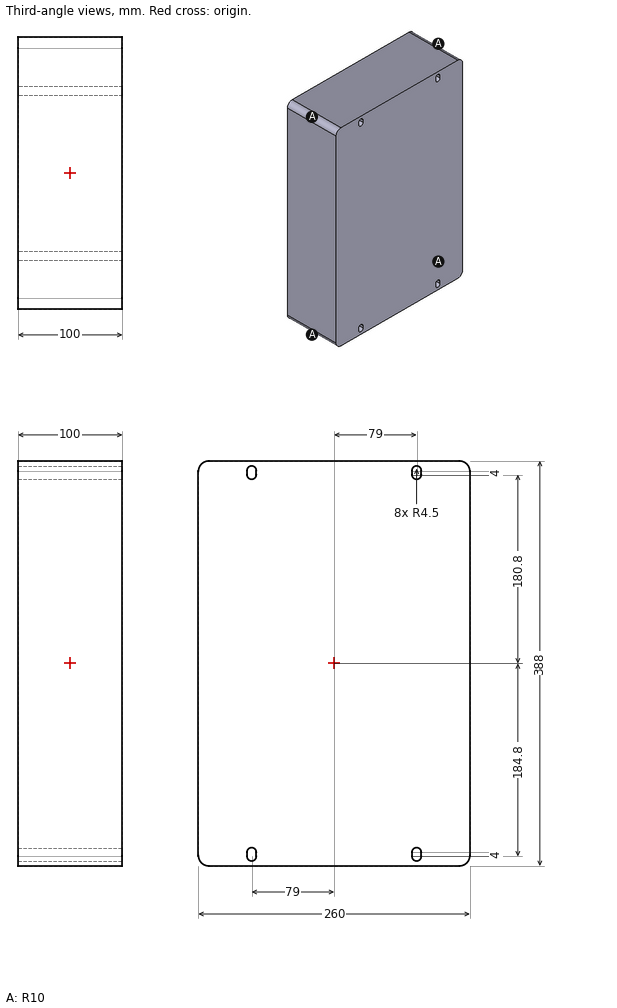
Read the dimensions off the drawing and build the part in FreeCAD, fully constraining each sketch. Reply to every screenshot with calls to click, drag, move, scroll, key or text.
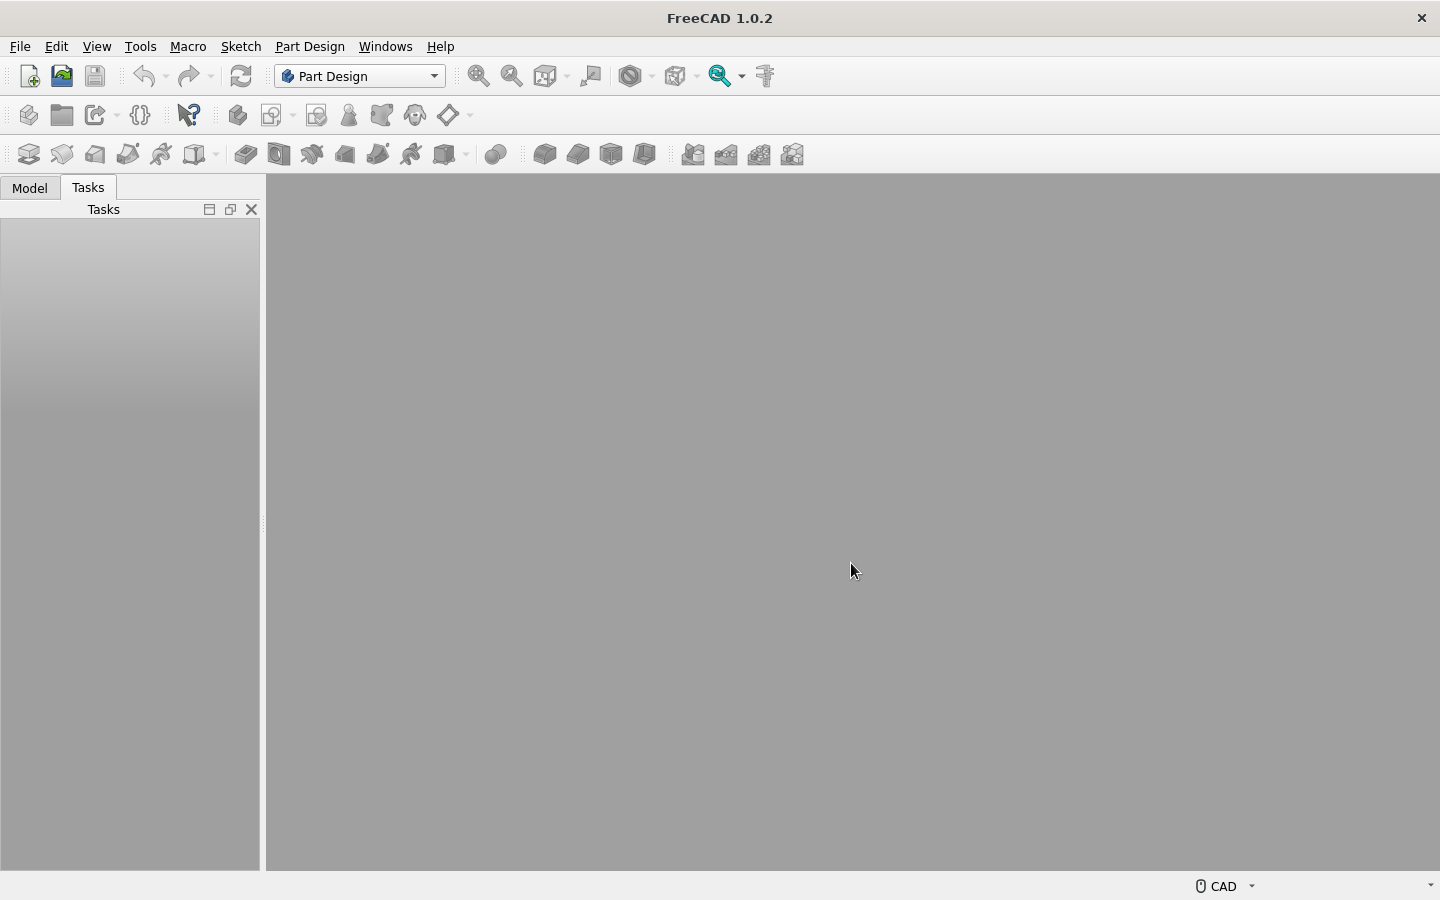
click(29, 76)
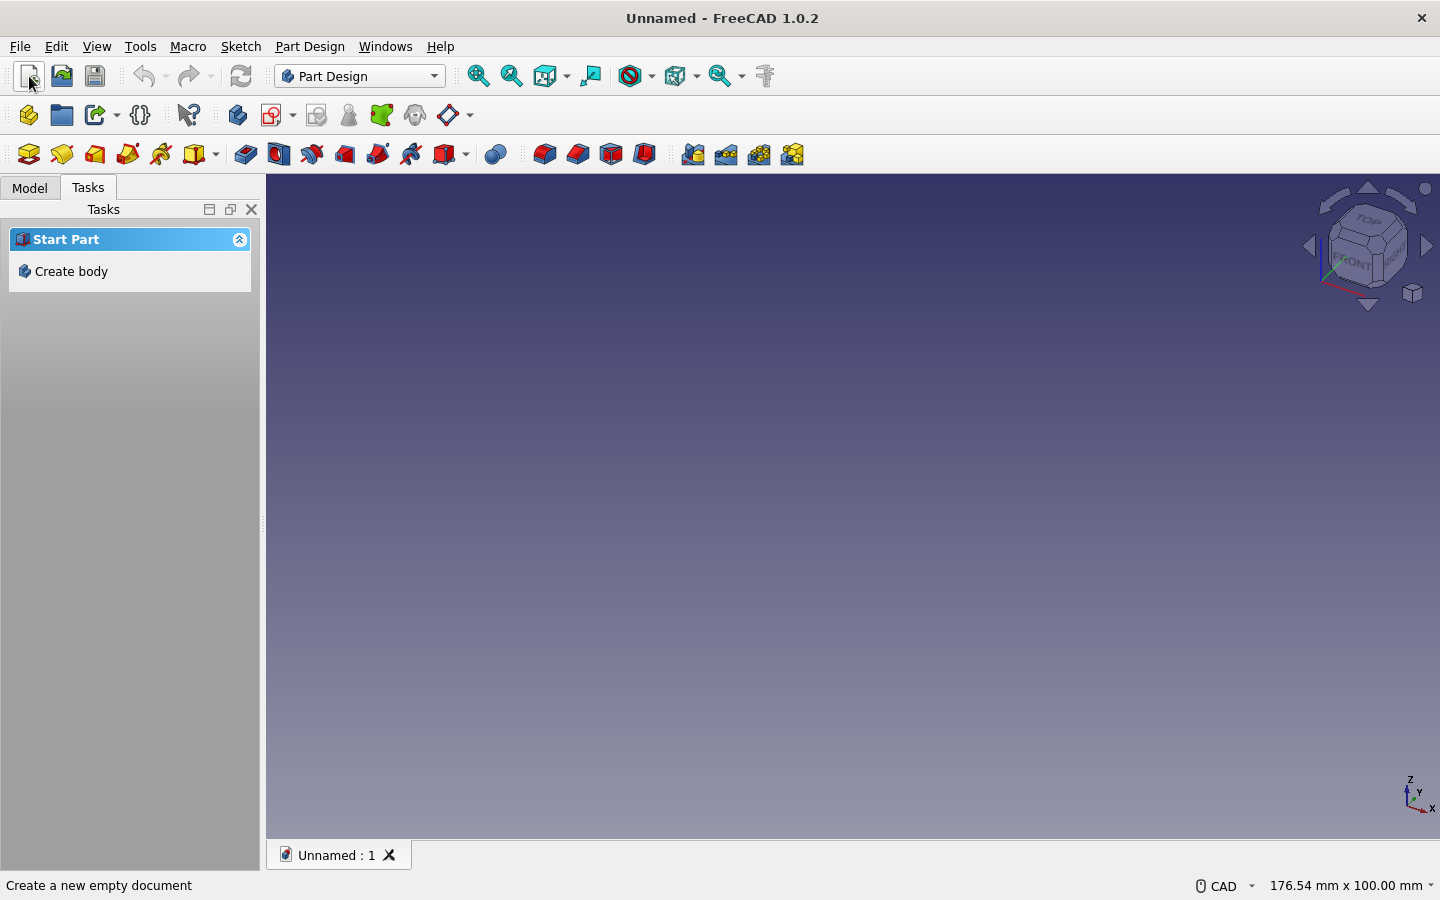
click(270, 116)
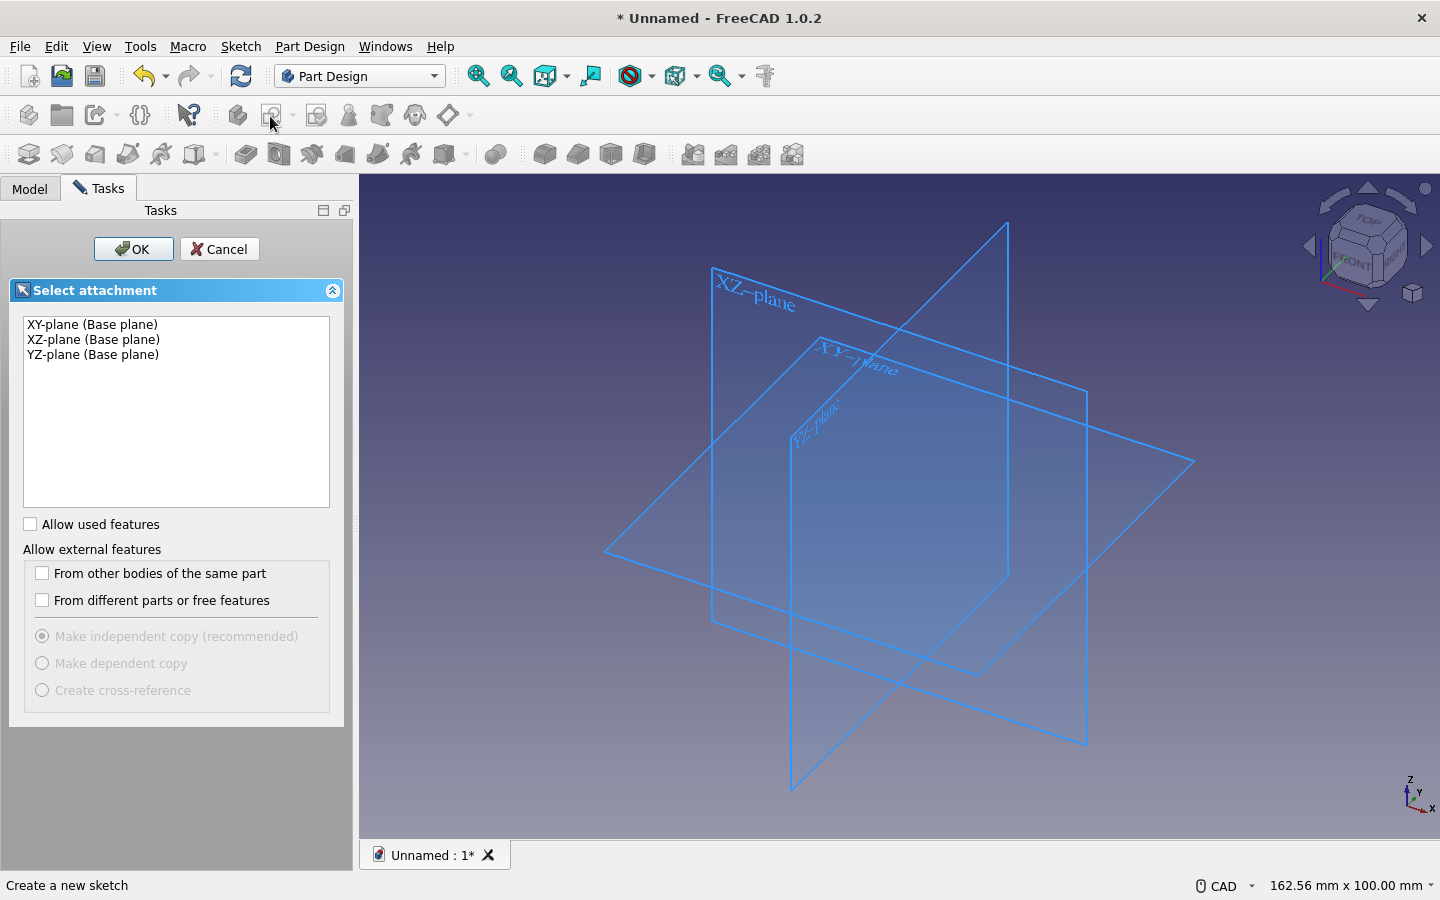
click(84, 354)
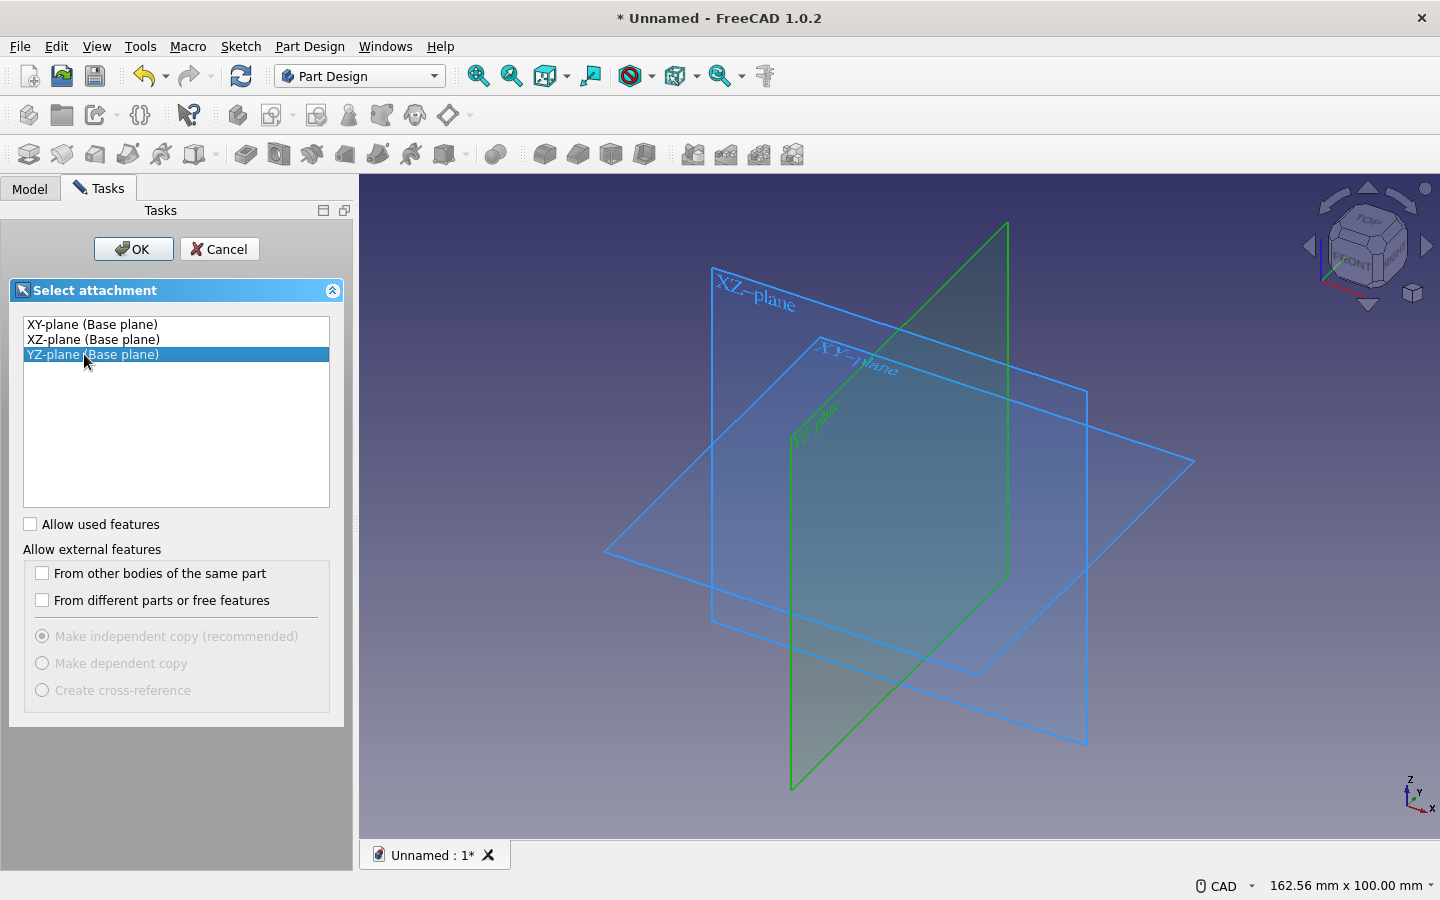
click(134, 249)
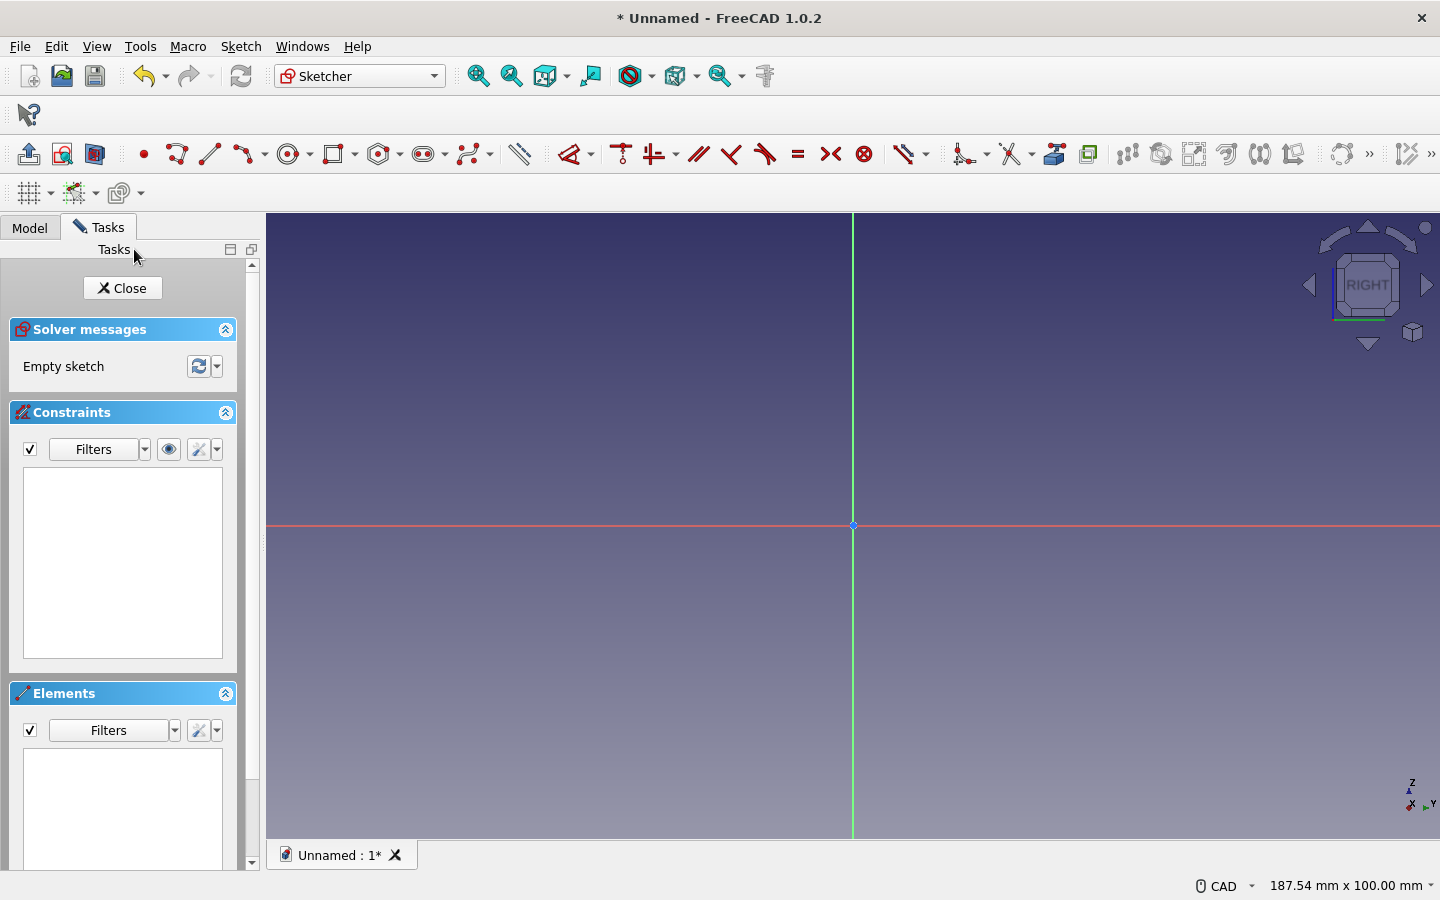
scroll(771, 526, down, 9)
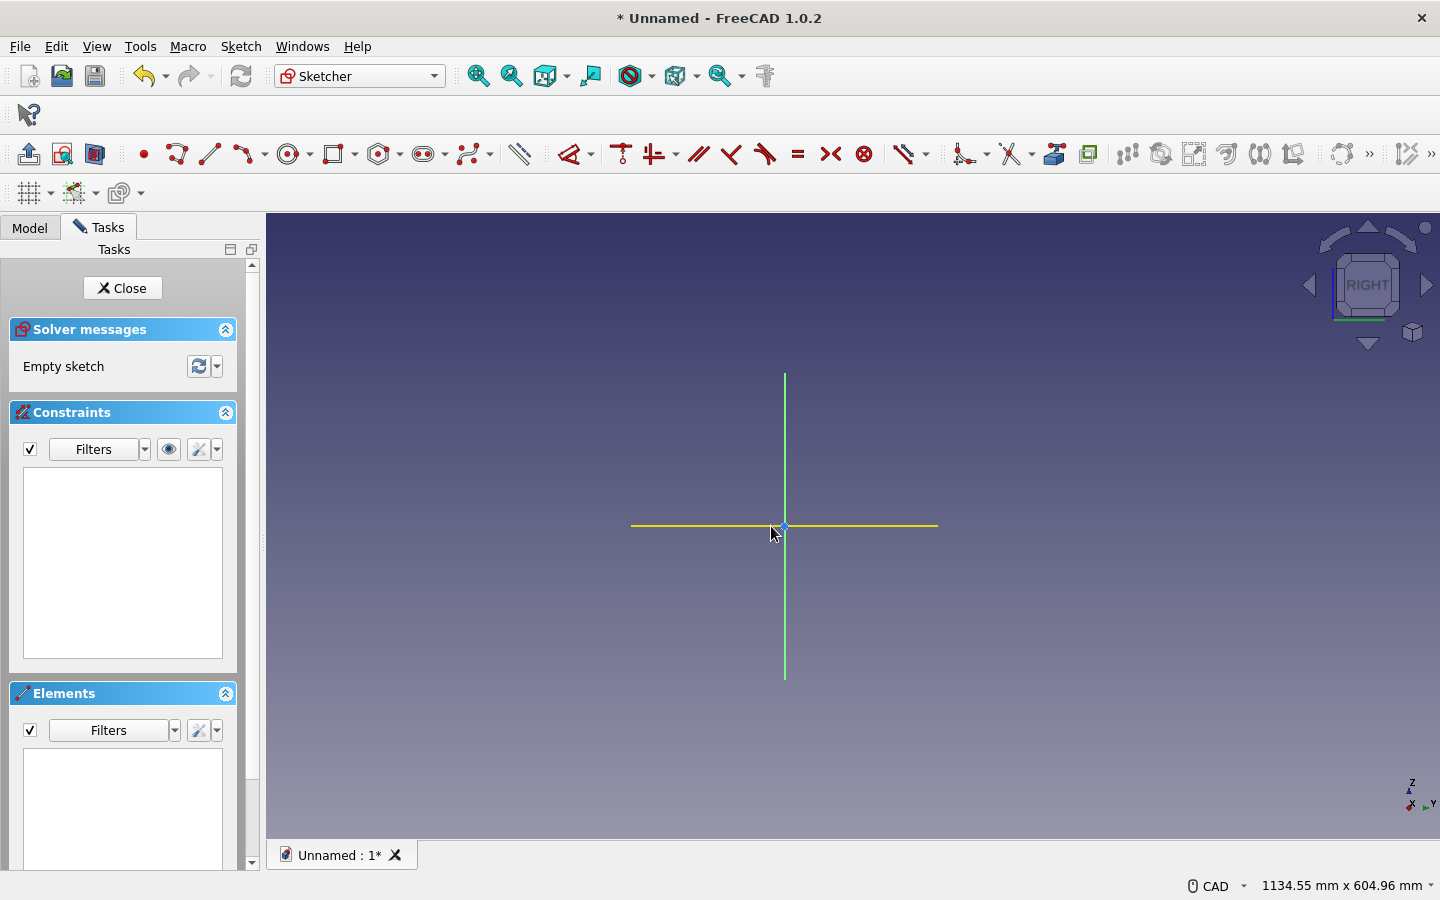
key(g)
key(v)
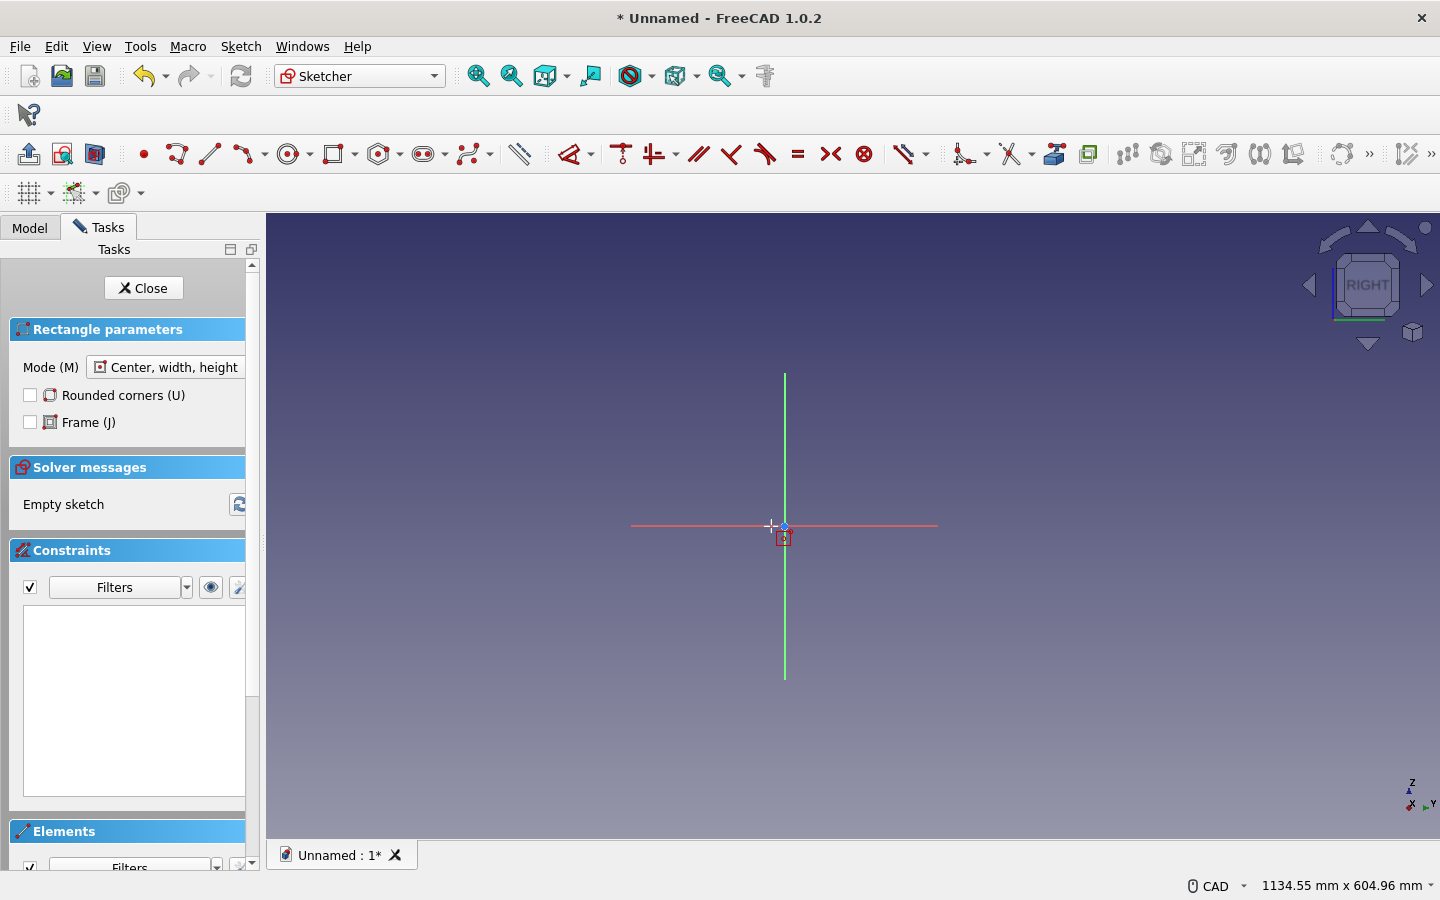
click(785, 526)
move(919, 326)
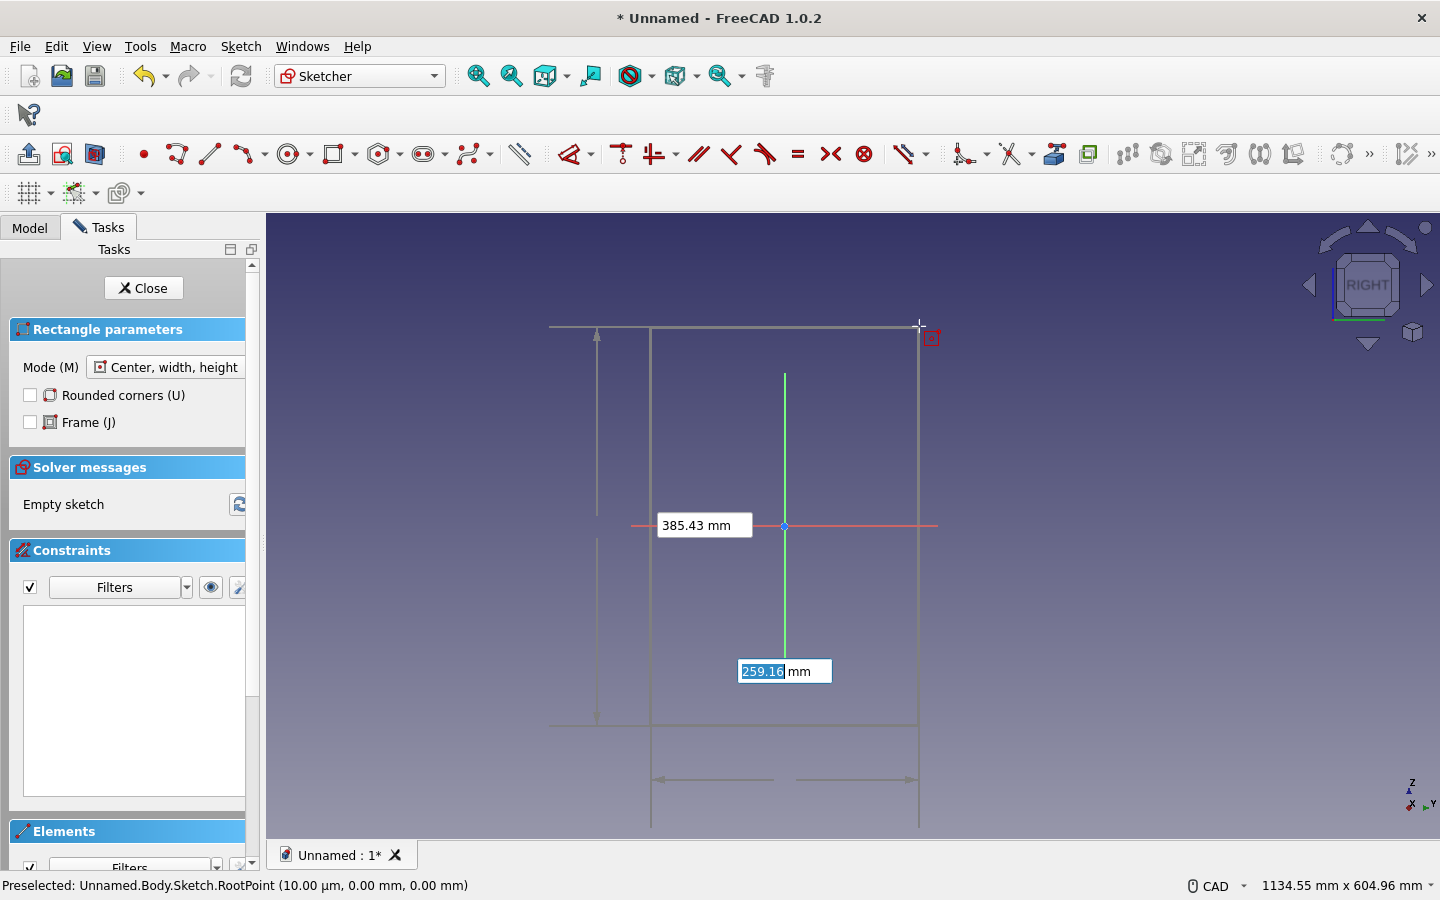
text(260)
key(Tab)
text(388)
key(Return)
key(Escape)